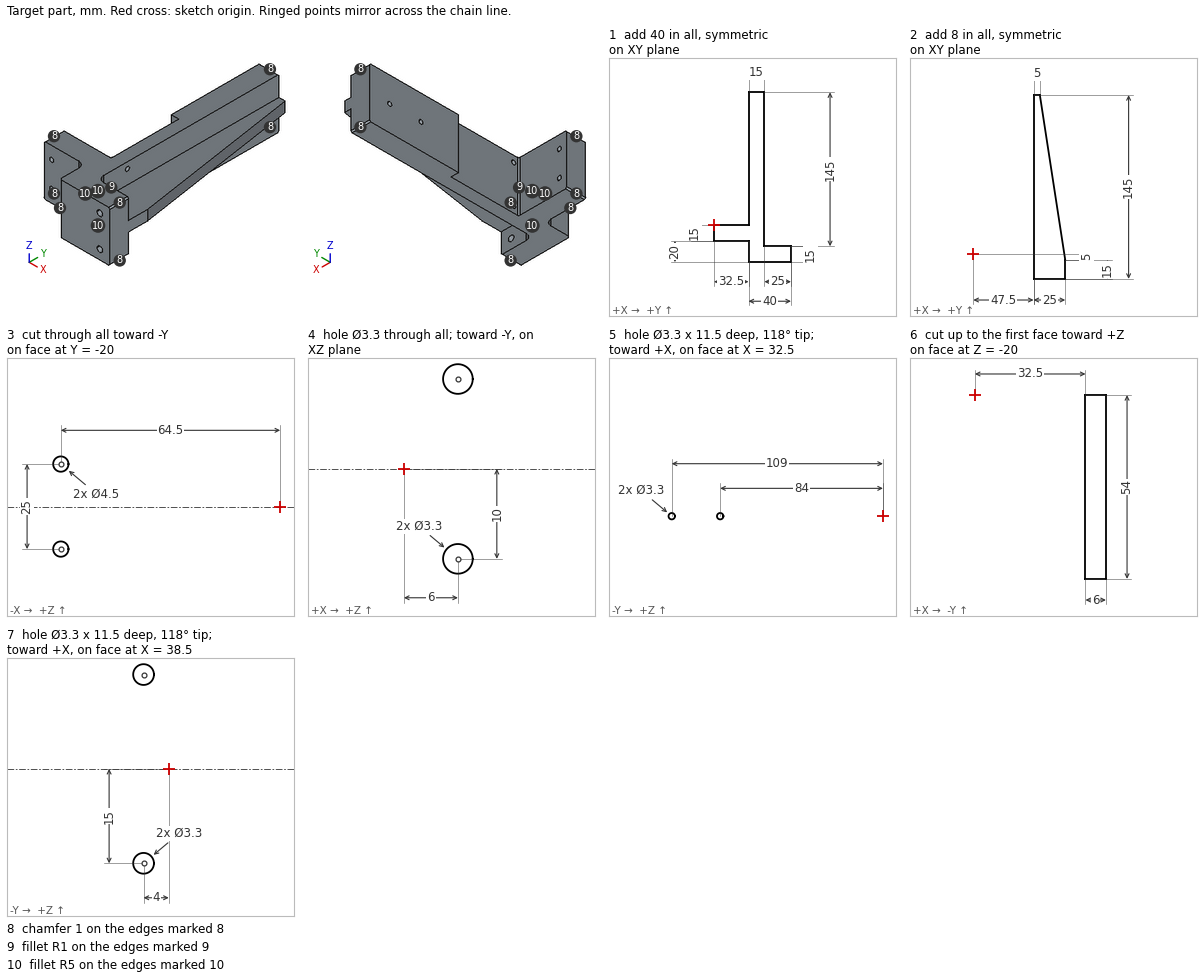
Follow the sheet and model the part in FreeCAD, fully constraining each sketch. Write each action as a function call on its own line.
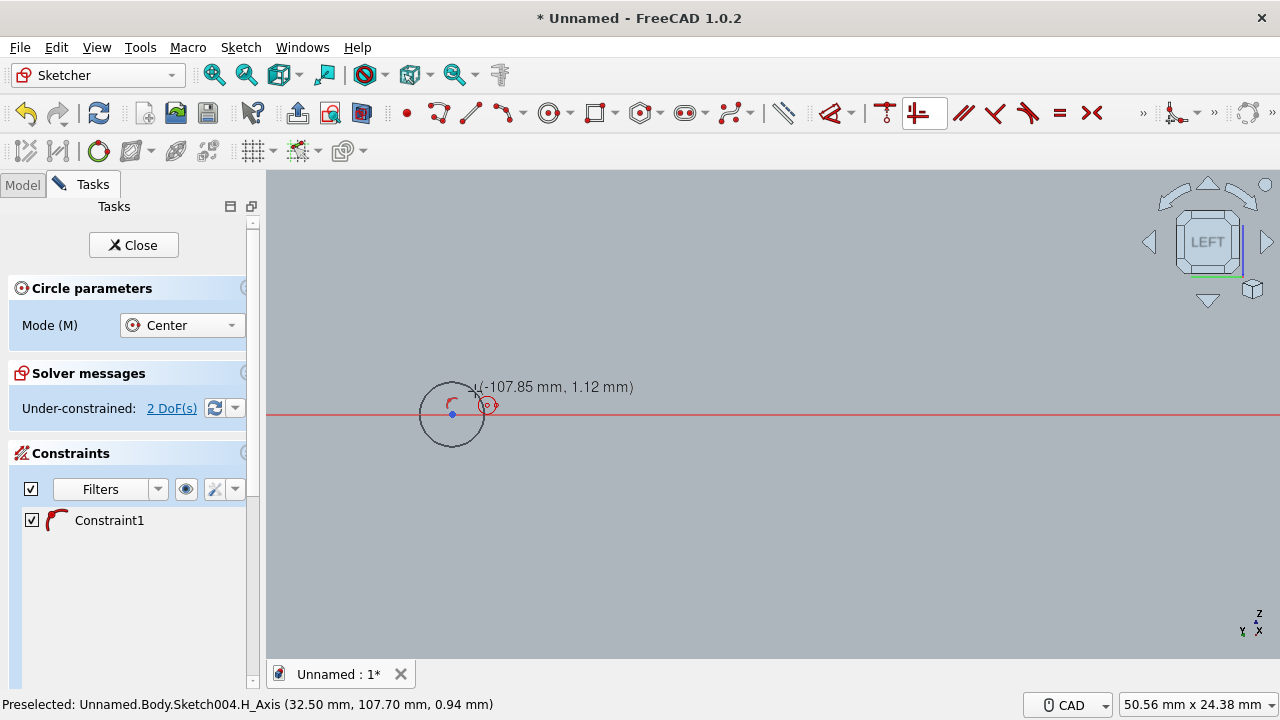
click(953, 414)
click(977, 391)
key(Escape)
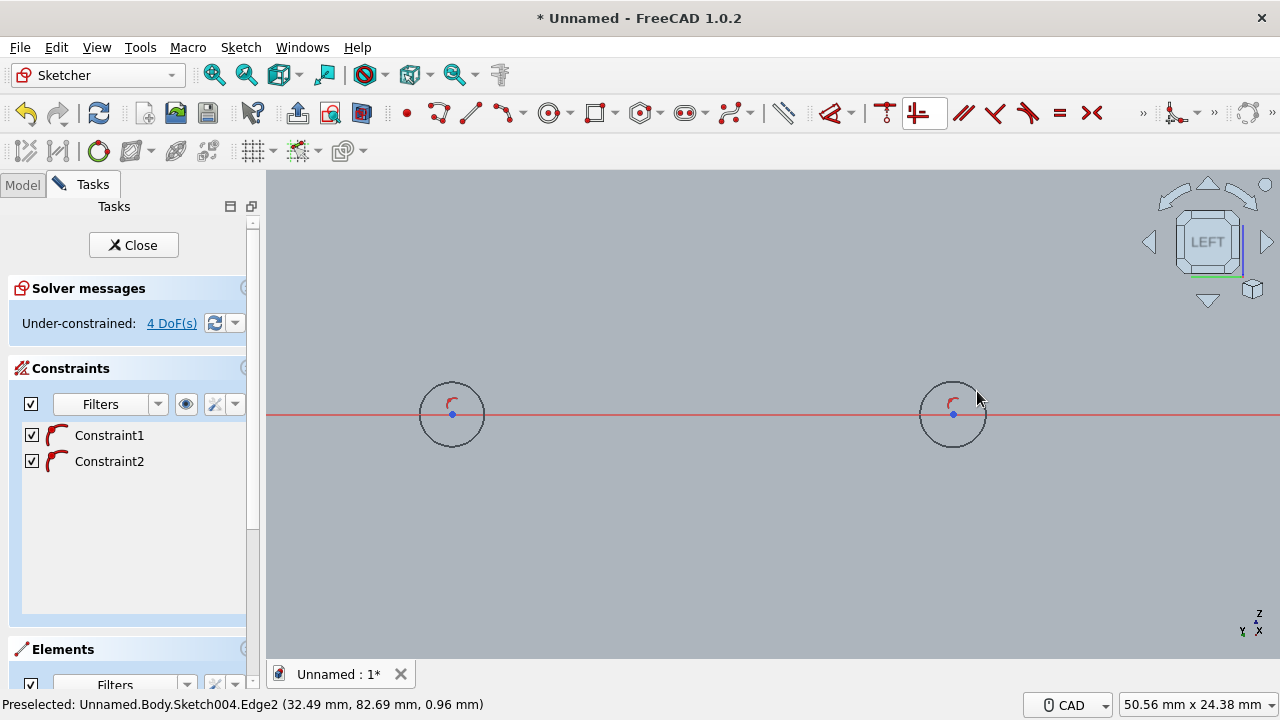
click(475, 392)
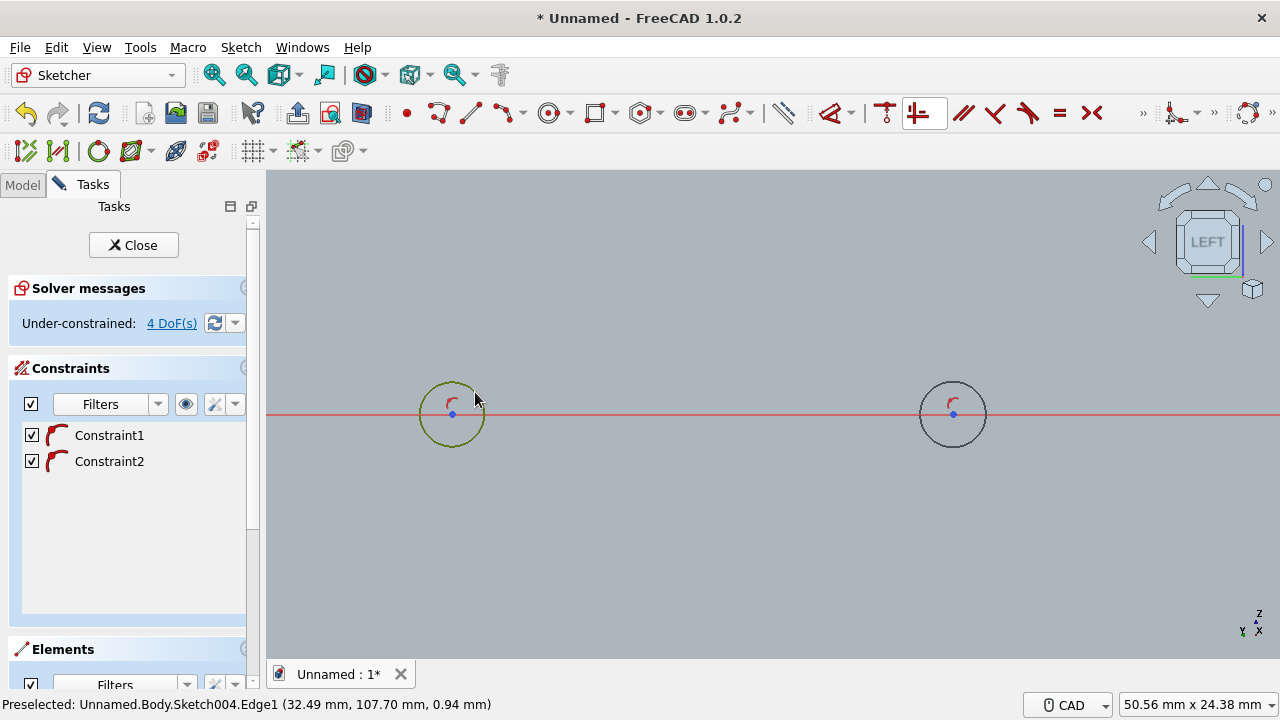
click(976, 391)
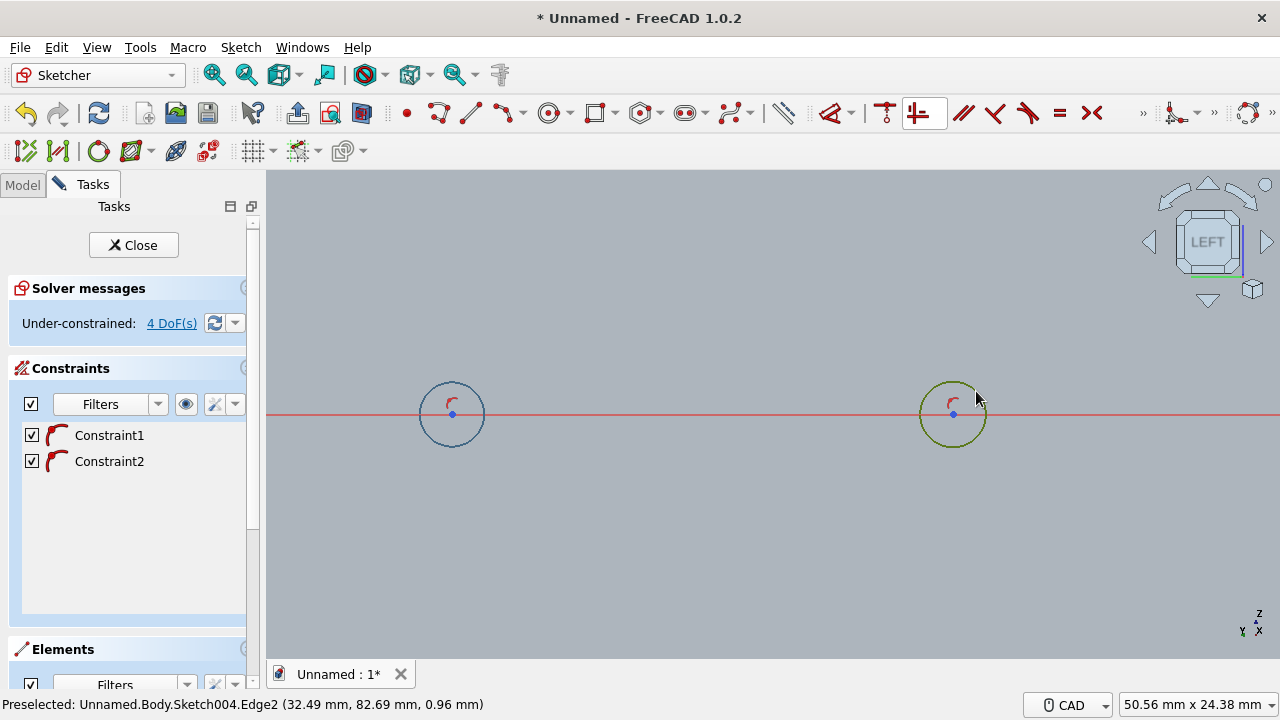
click(1060, 114)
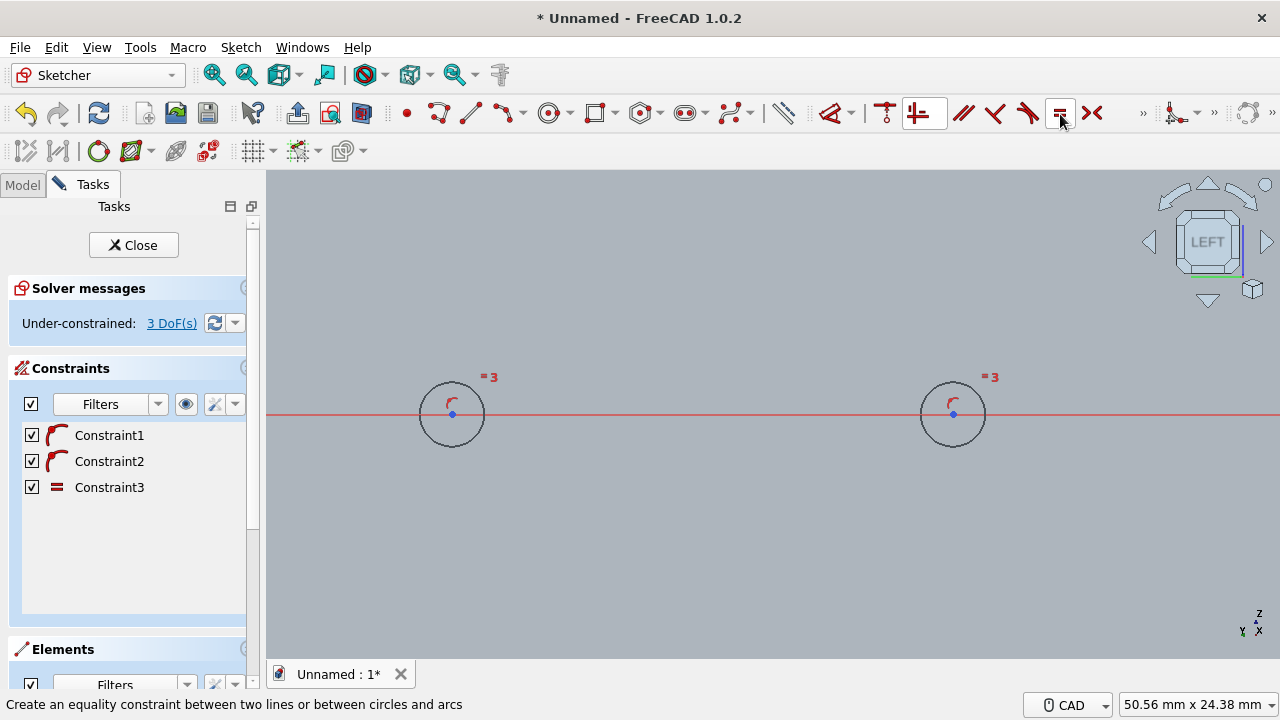
click(830, 114)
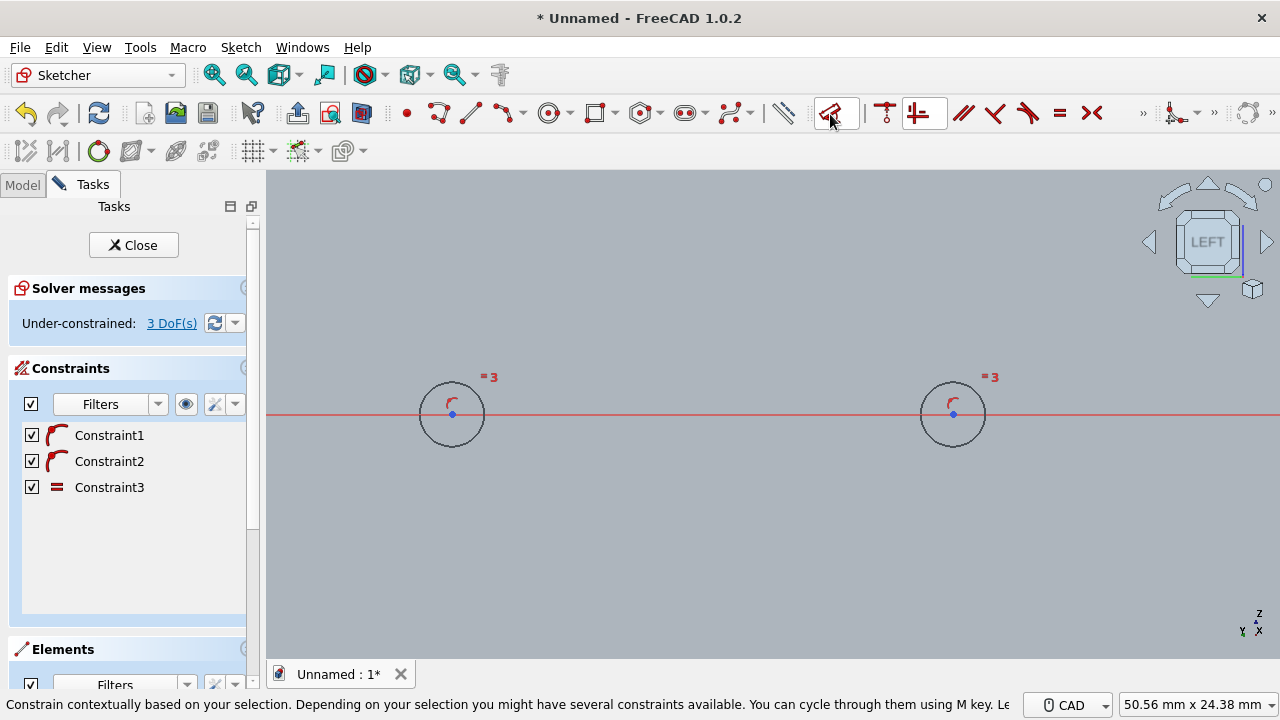
click(475, 392)
click(498, 370)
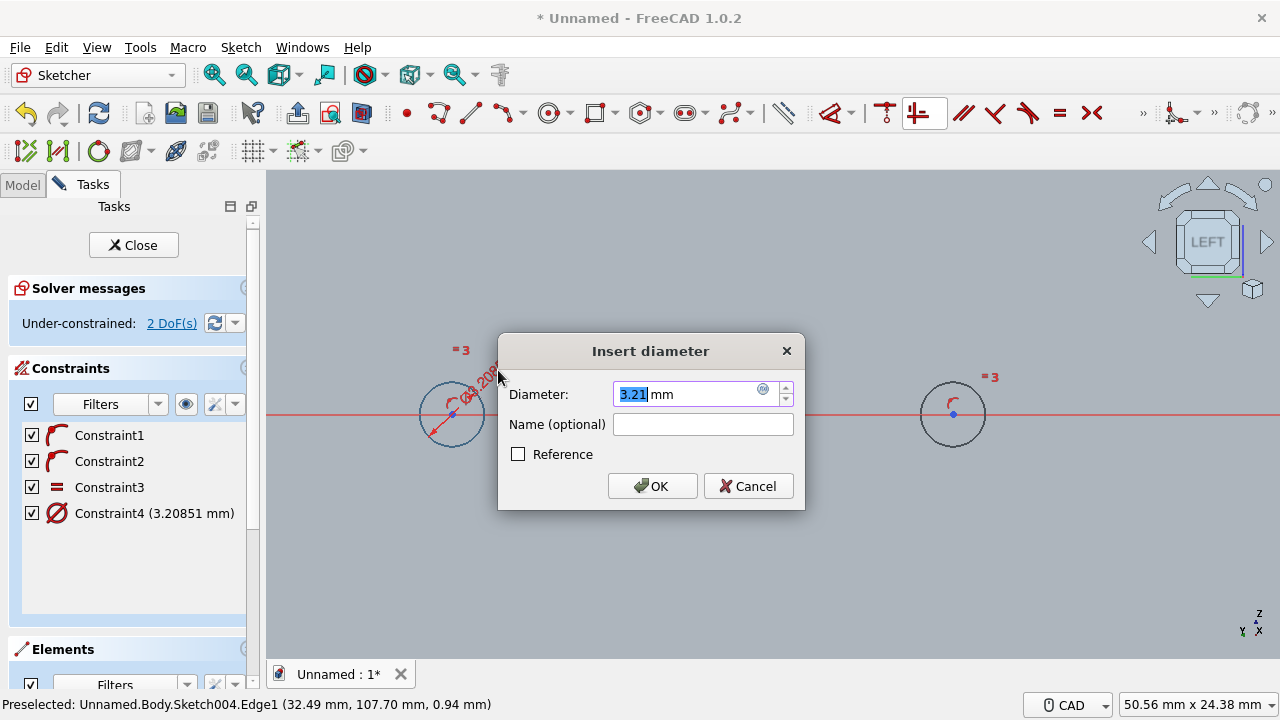
text(3.3)
key(Return)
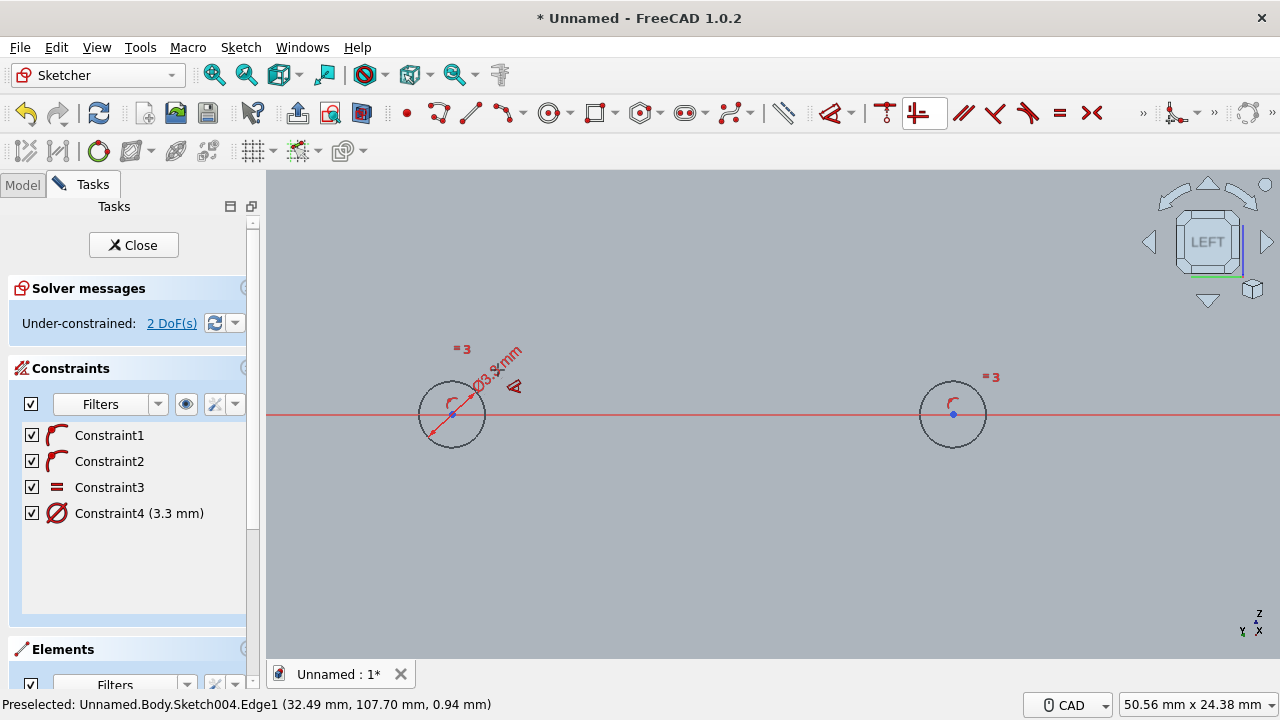
click(953, 414)
click(1034, 448)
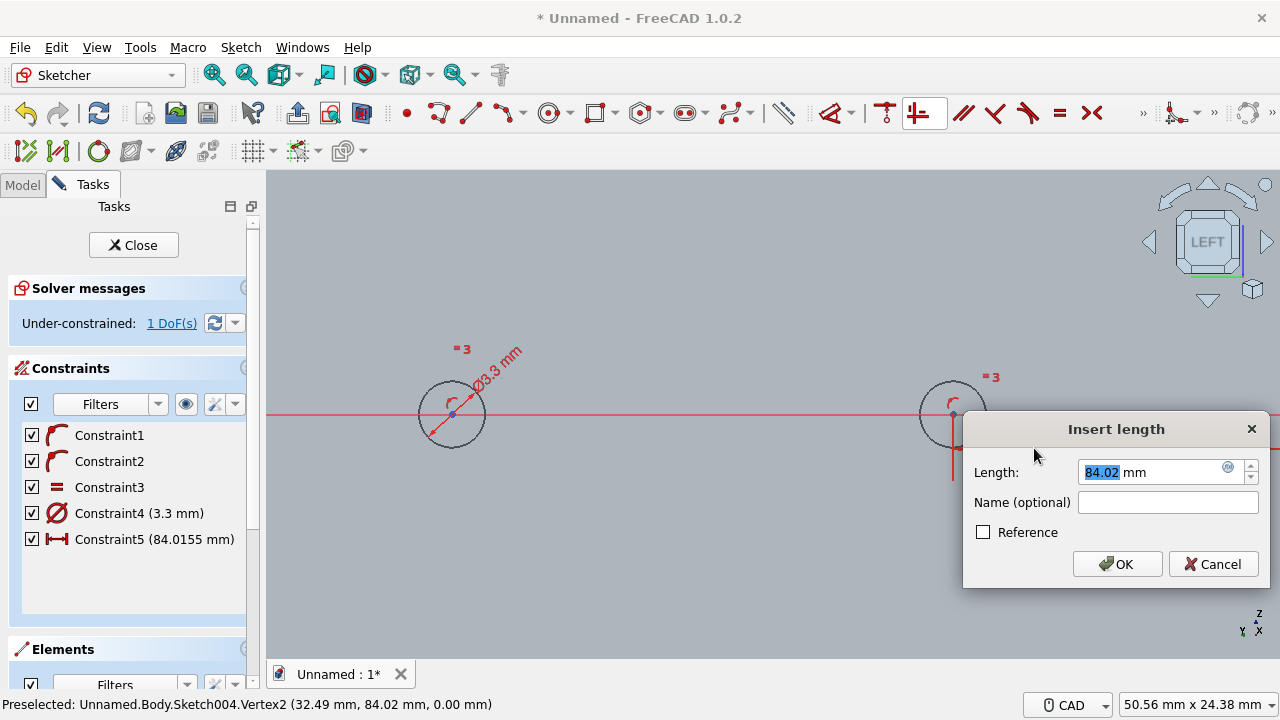
text(84)
key(Return)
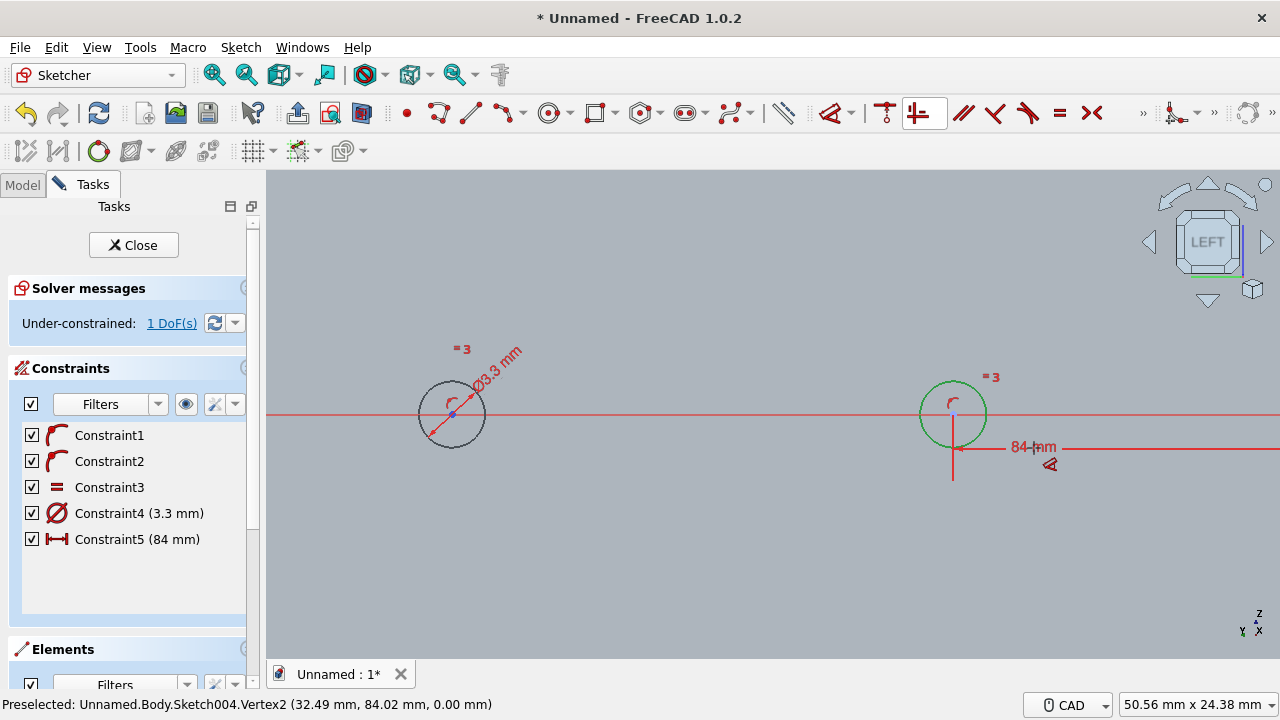
click(452, 414)
click(784, 448)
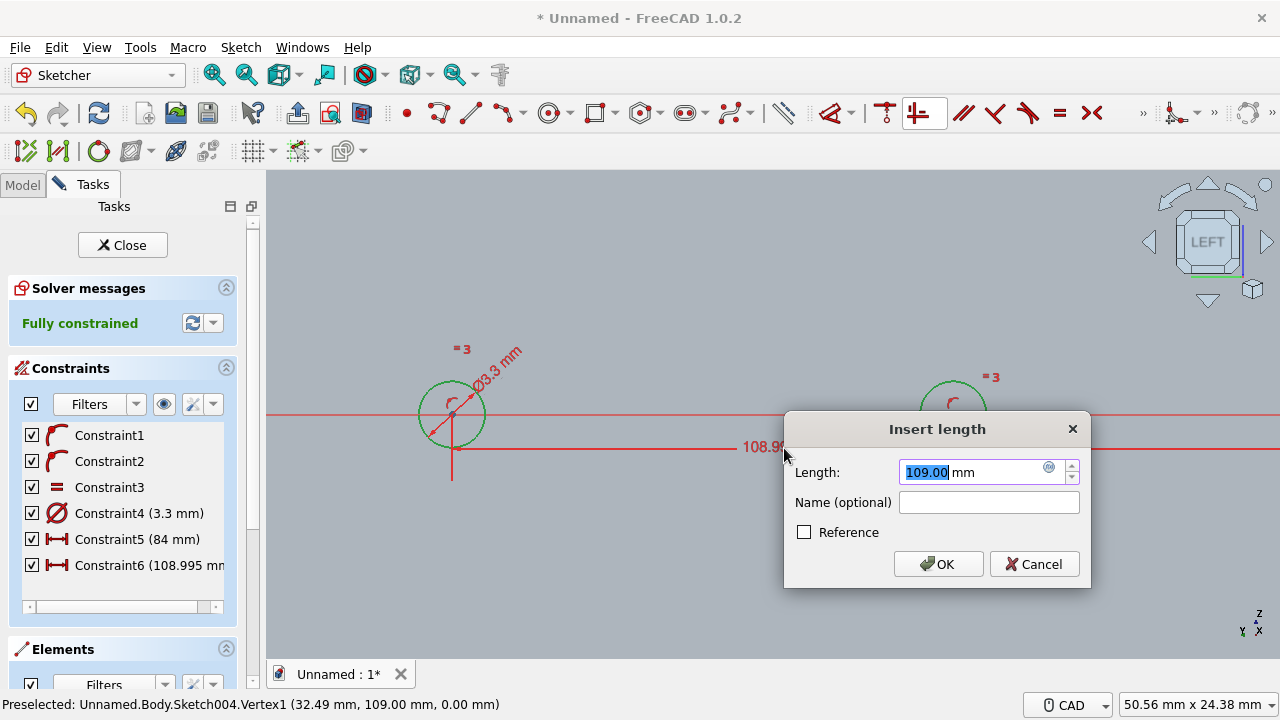
text(109)
key(Return)
key(Escape)